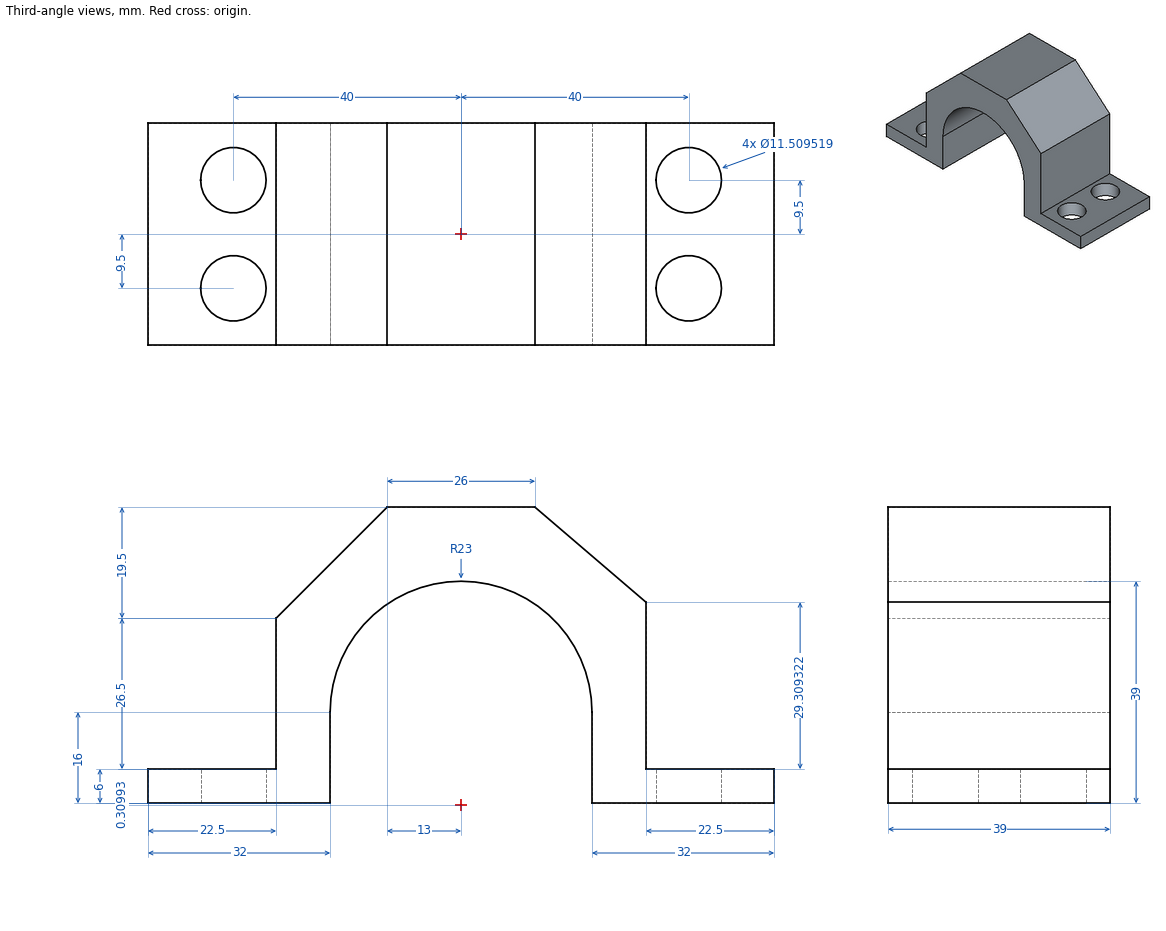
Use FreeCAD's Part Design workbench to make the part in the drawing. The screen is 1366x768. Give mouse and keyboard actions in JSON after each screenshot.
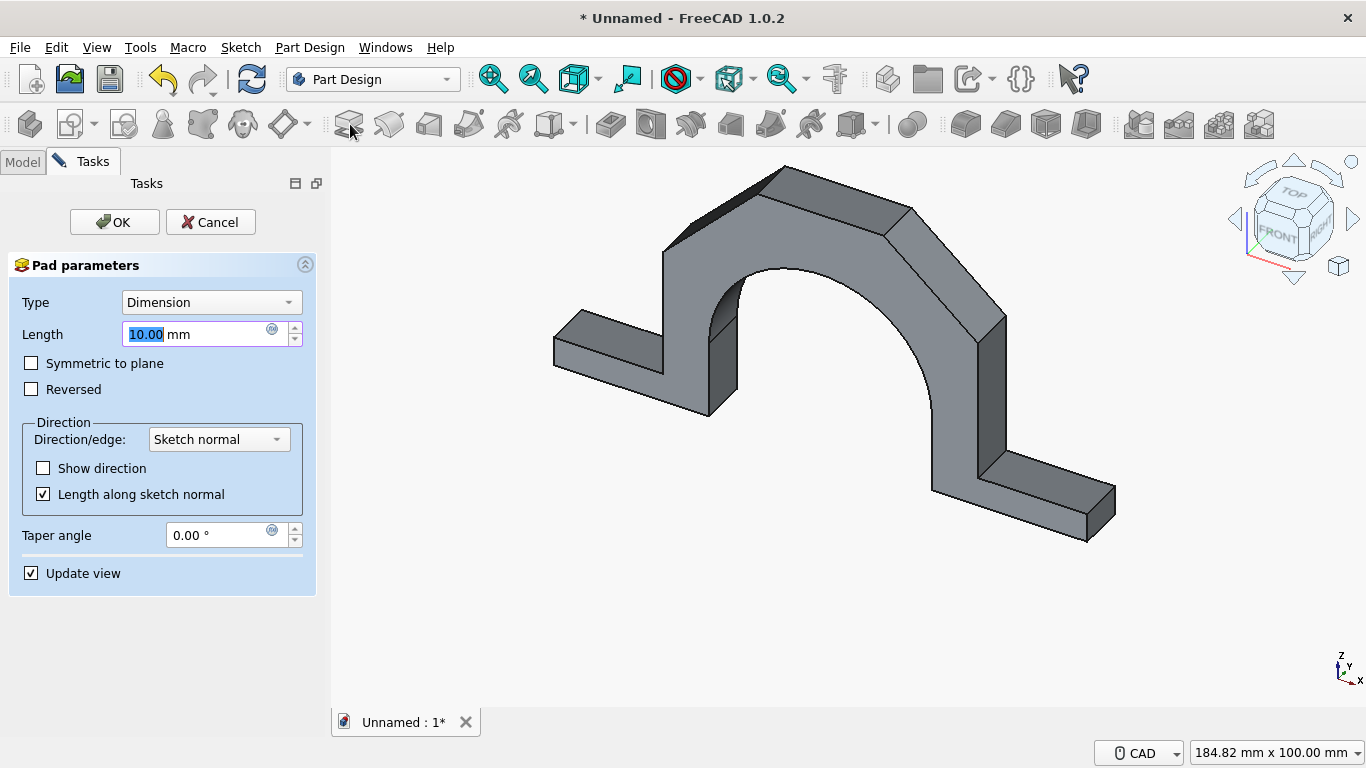
{"action": "type", "text": "39"}
{"action": "key", "text": "Tab"}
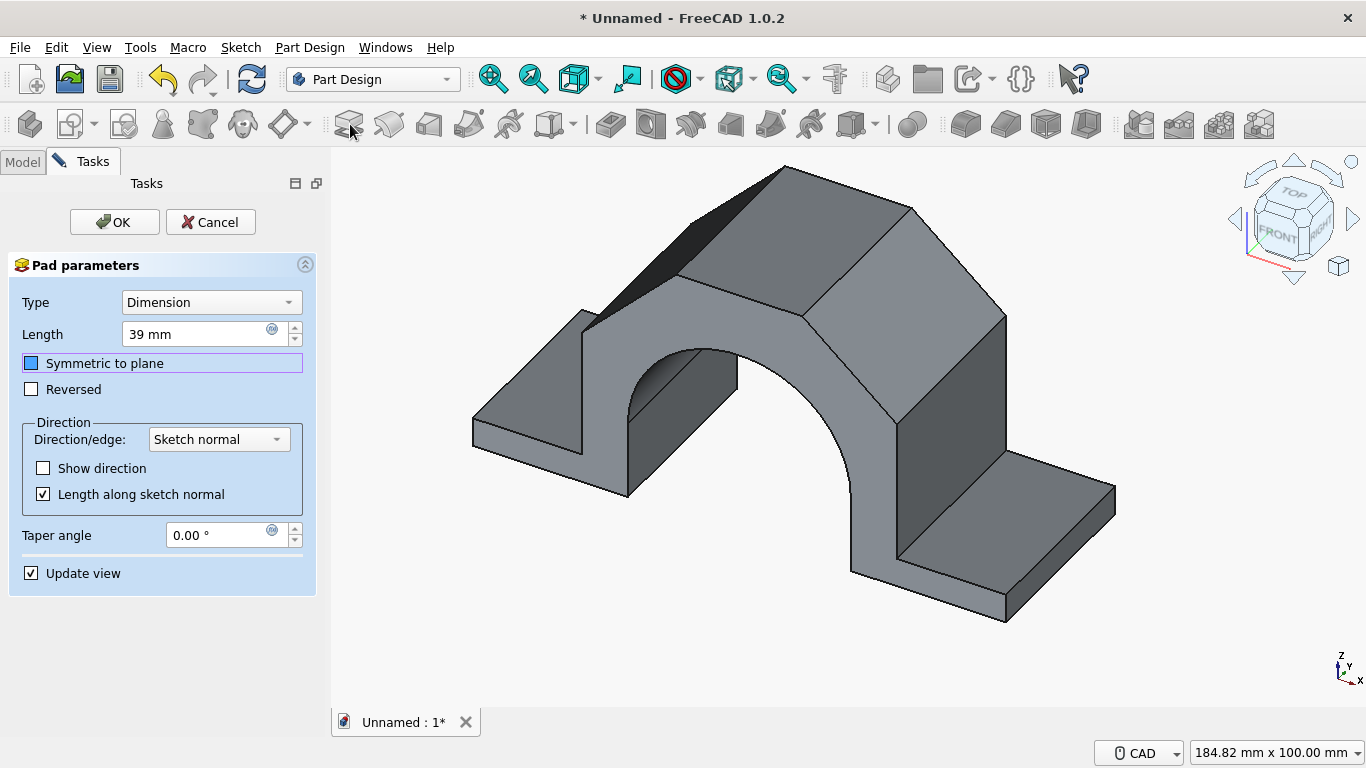
{"action": "left_click", "coordinate": [30, 363]}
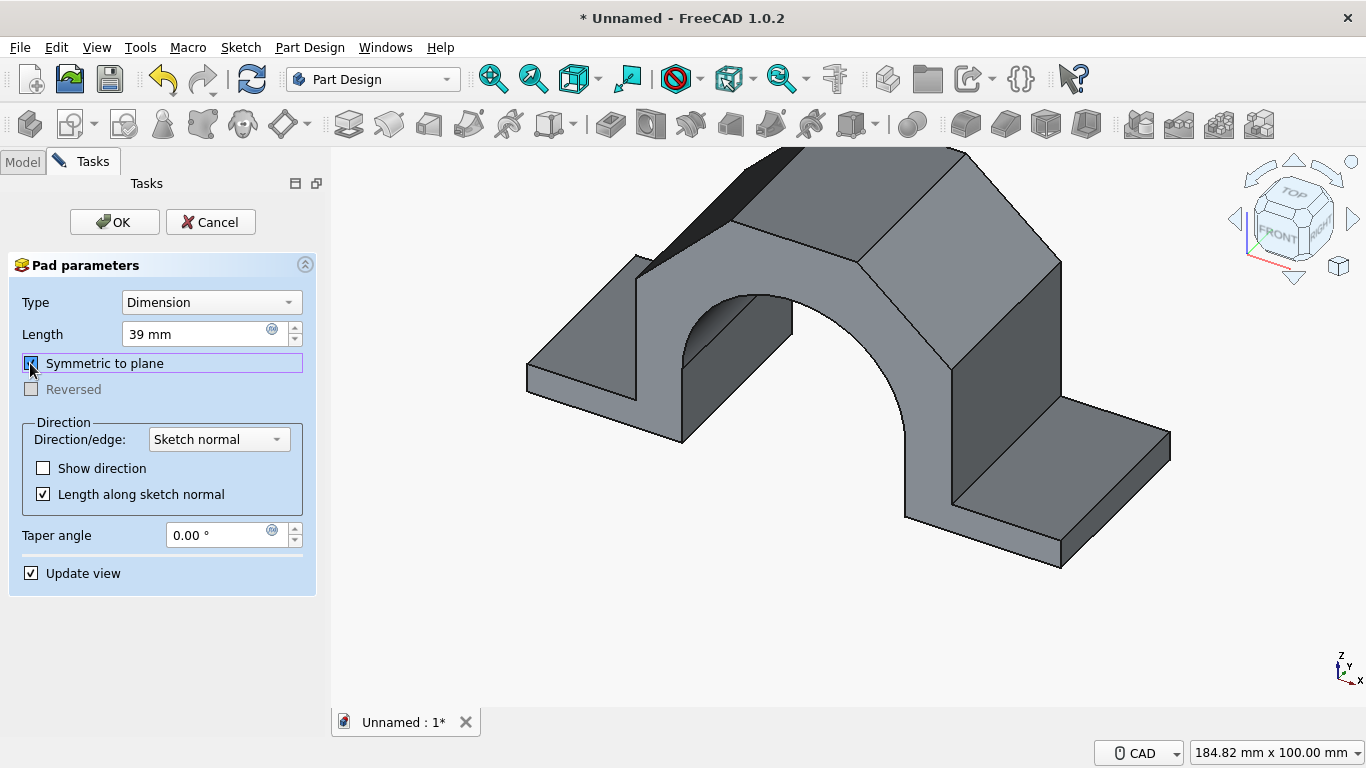
{"action": "left_click", "coordinate": [115, 222]}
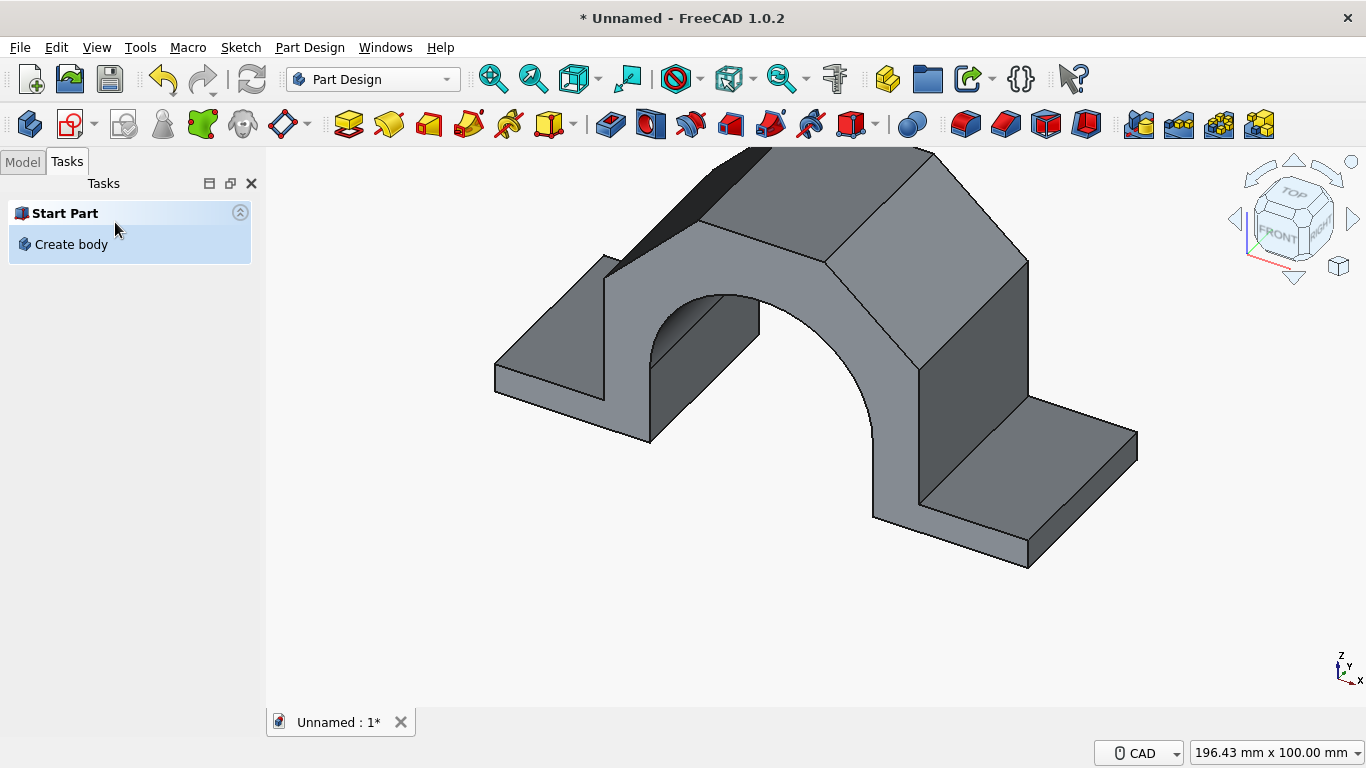
{"action": "key", "text": "v f"}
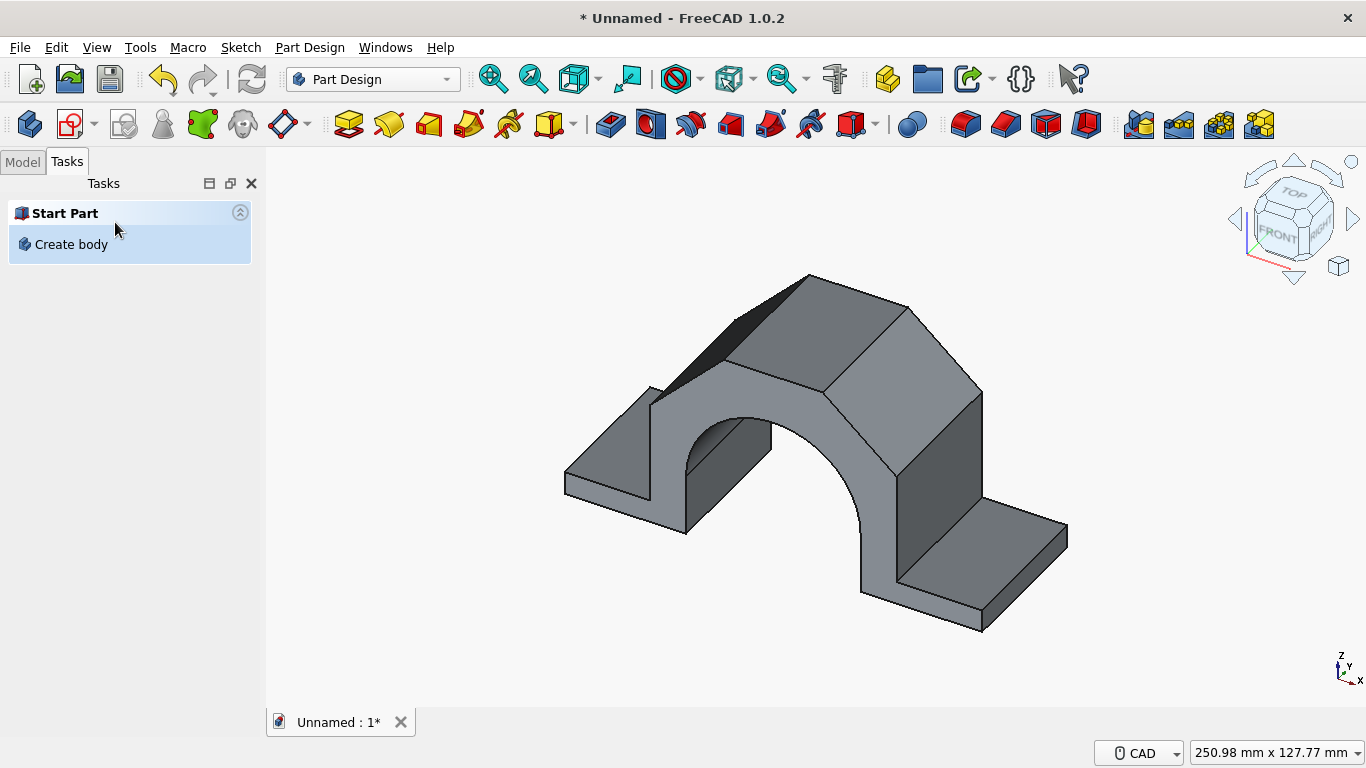
{"action": "key", "text": "5"}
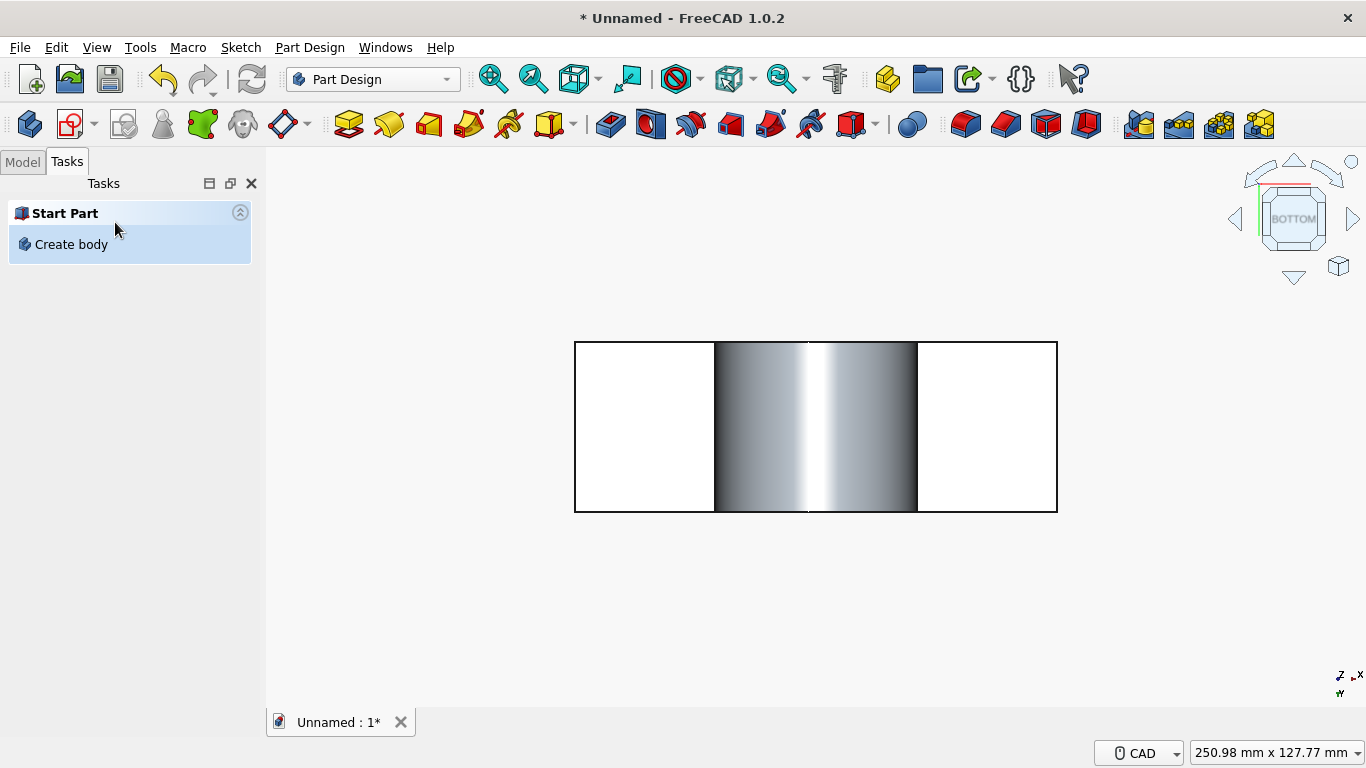
{"action": "key", "text": "v f"}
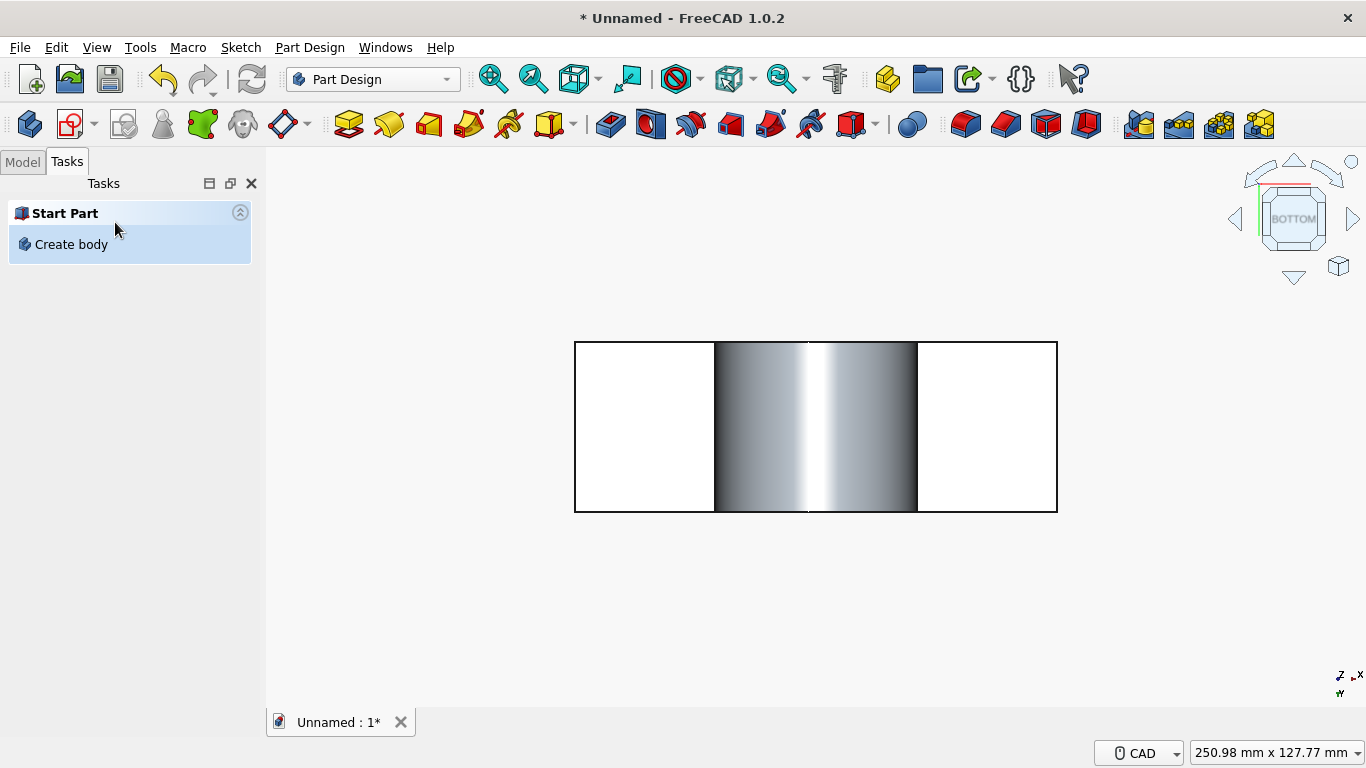
{"action": "left_click", "coordinate": [645, 426]}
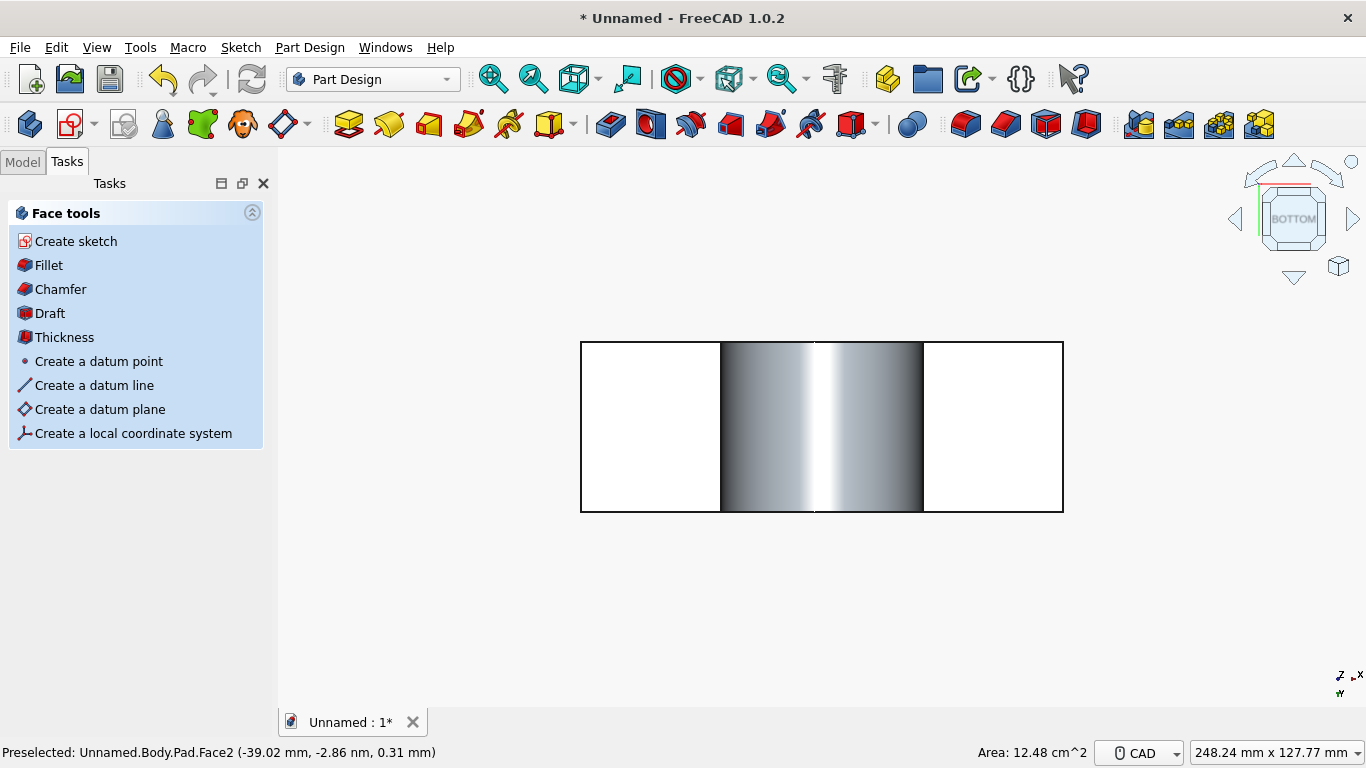
{"action": "left_click", "coordinate": [70, 124]}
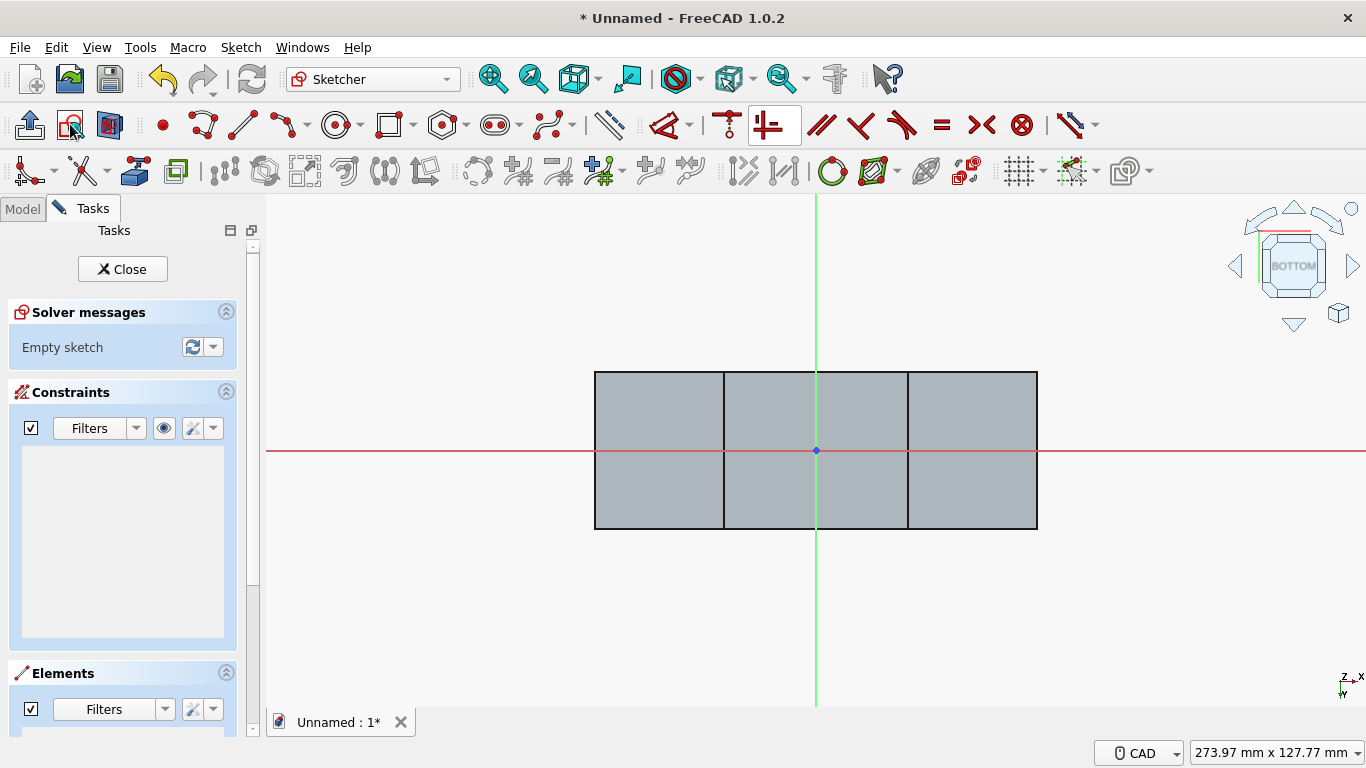
{"action": "scroll", "coordinate": [899, 451], "scroll_direction": "up", "scroll_amount": 3}